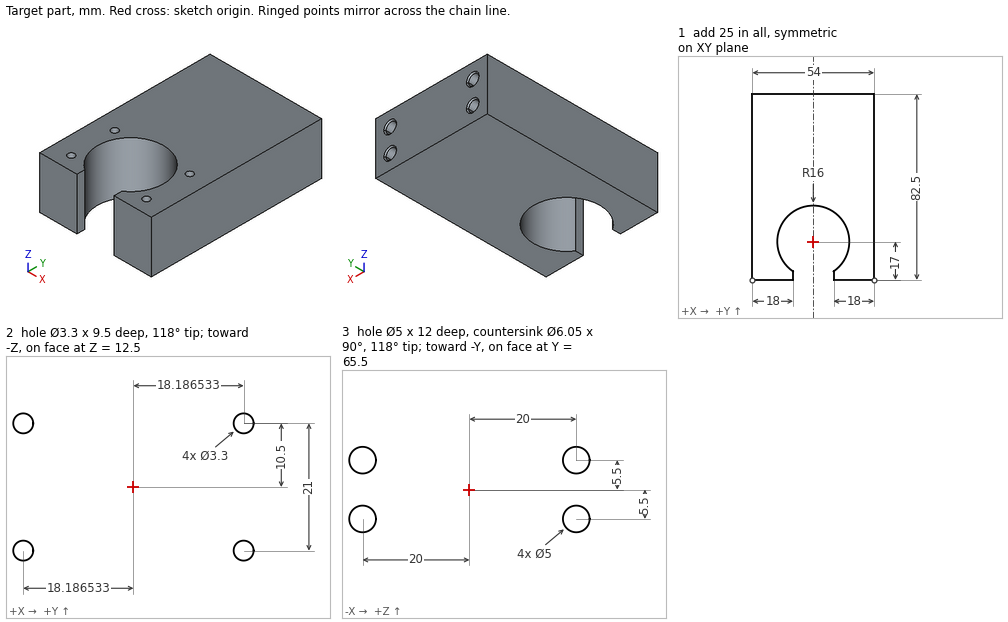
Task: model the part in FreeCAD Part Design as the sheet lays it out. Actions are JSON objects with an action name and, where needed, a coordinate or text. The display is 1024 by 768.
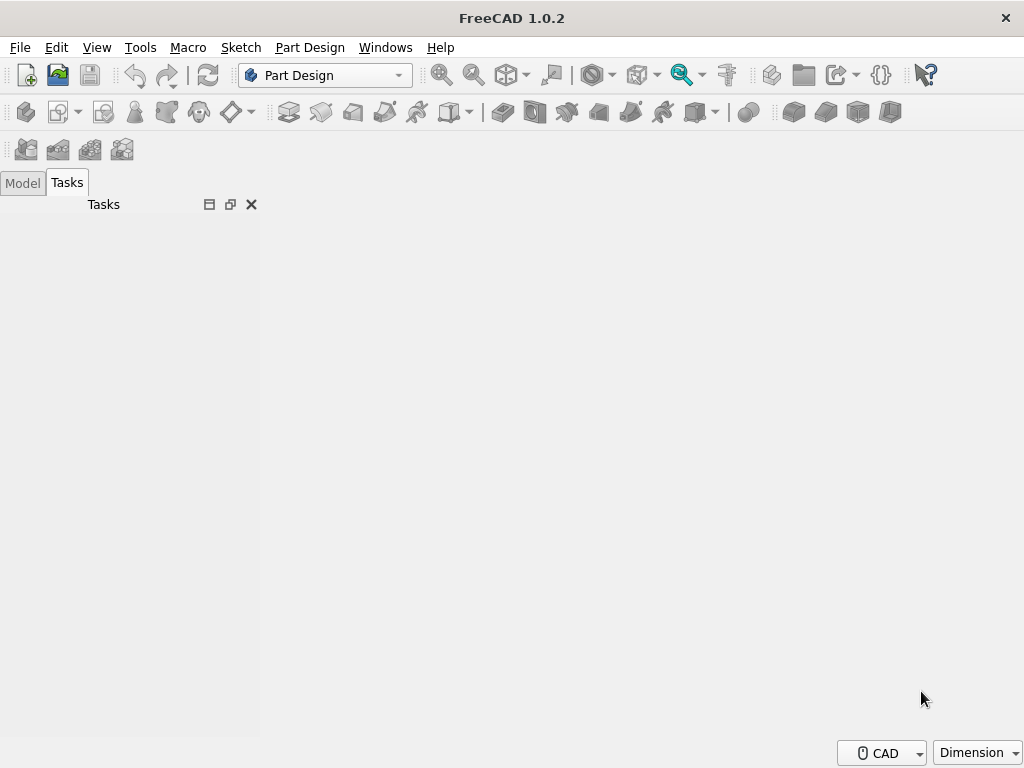
{"action": "left_click", "coordinate": [26, 76]}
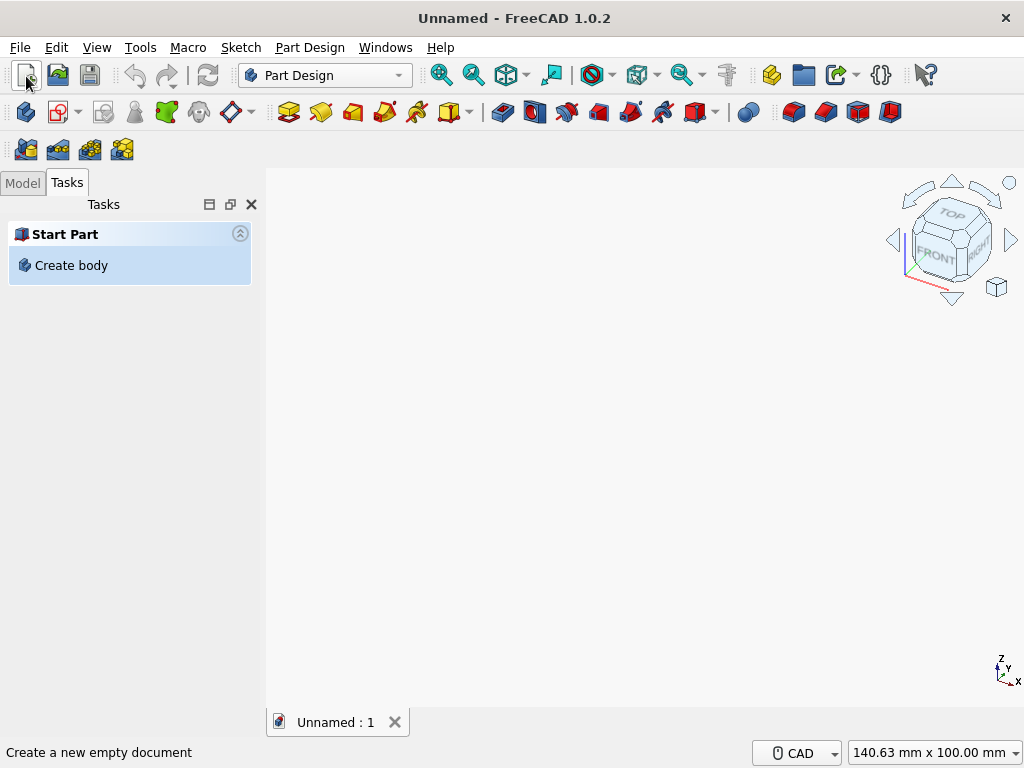
{"action": "left_click", "coordinate": [58, 112]}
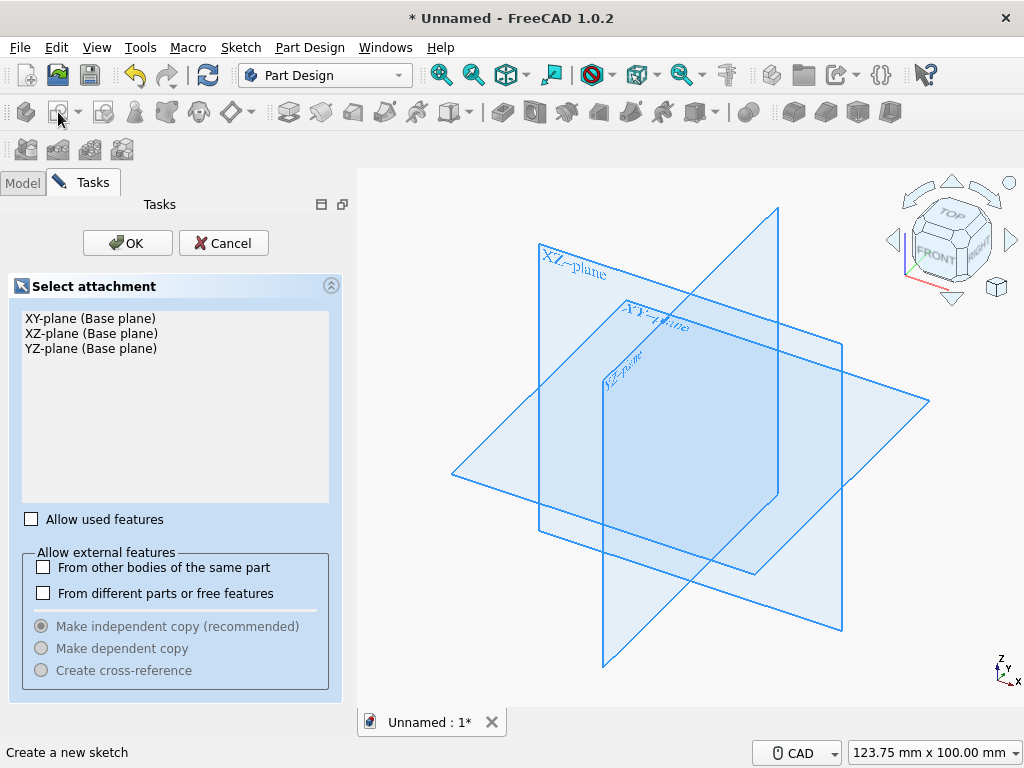
{"action": "left_click", "coordinate": [82, 318]}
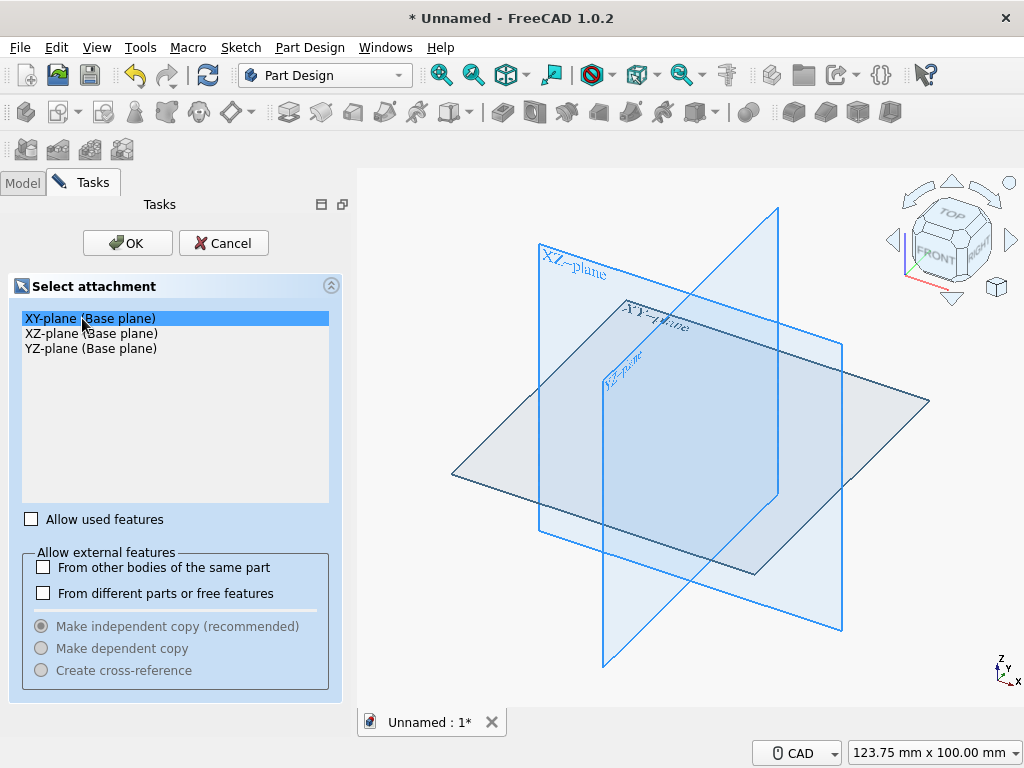
{"action": "left_click", "coordinate": [128, 243]}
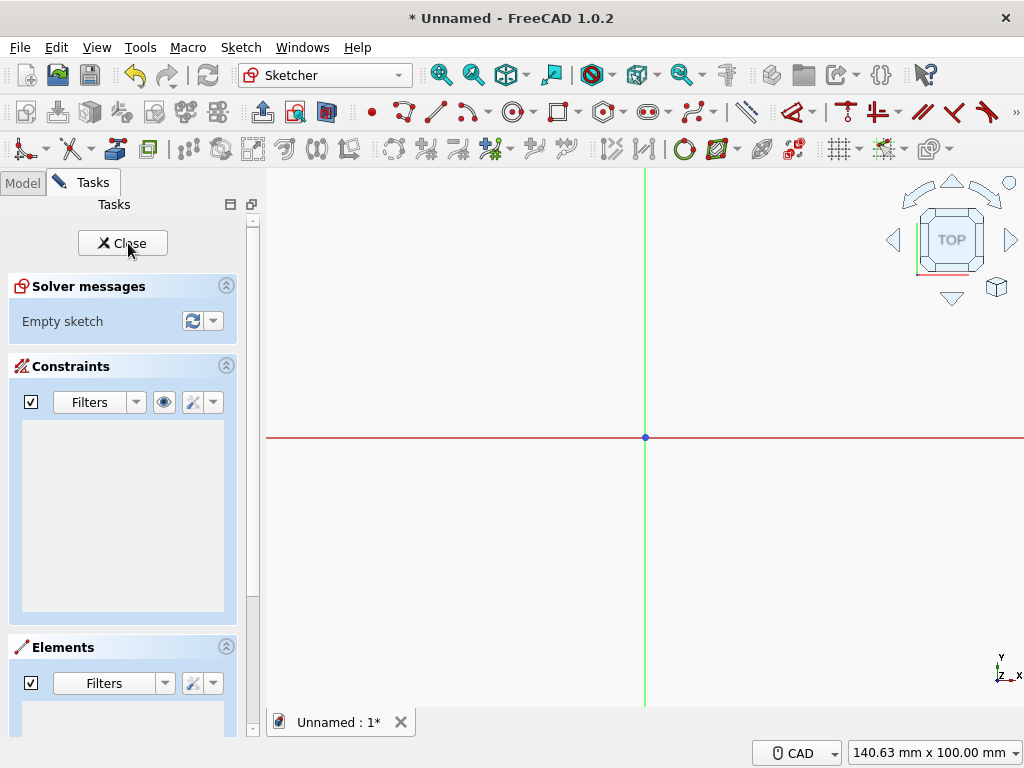
{"action": "scroll", "coordinate": [437, 679], "scroll_direction": "down", "scroll_amount": 2}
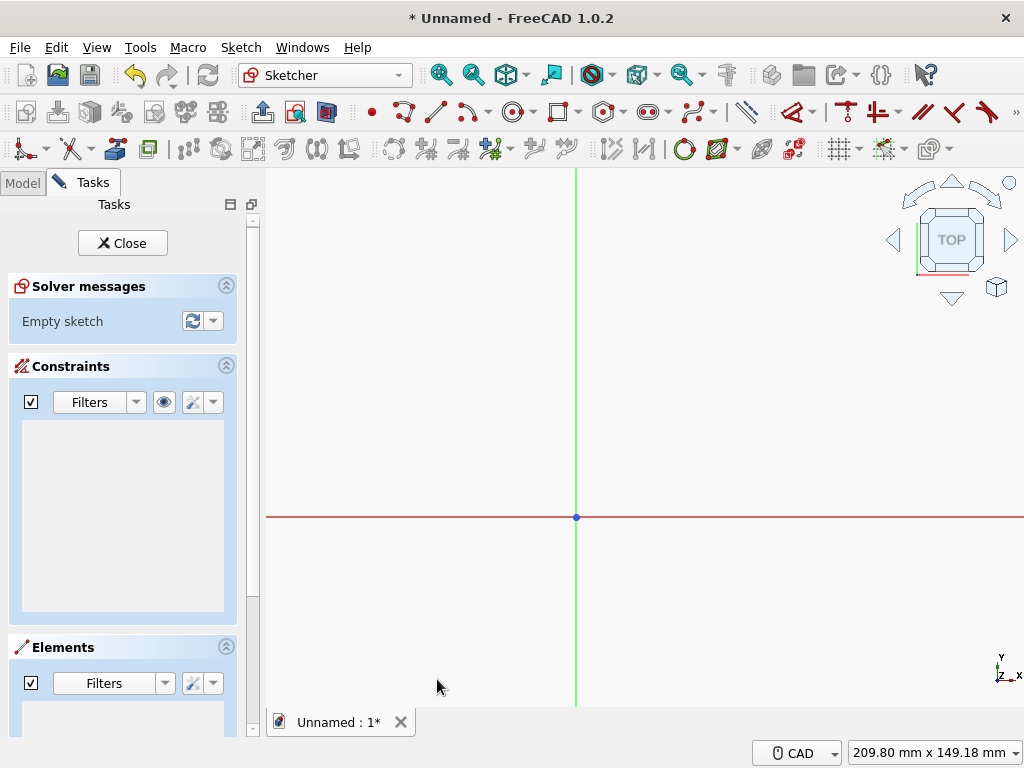
{"action": "left_click", "coordinate": [404, 112]}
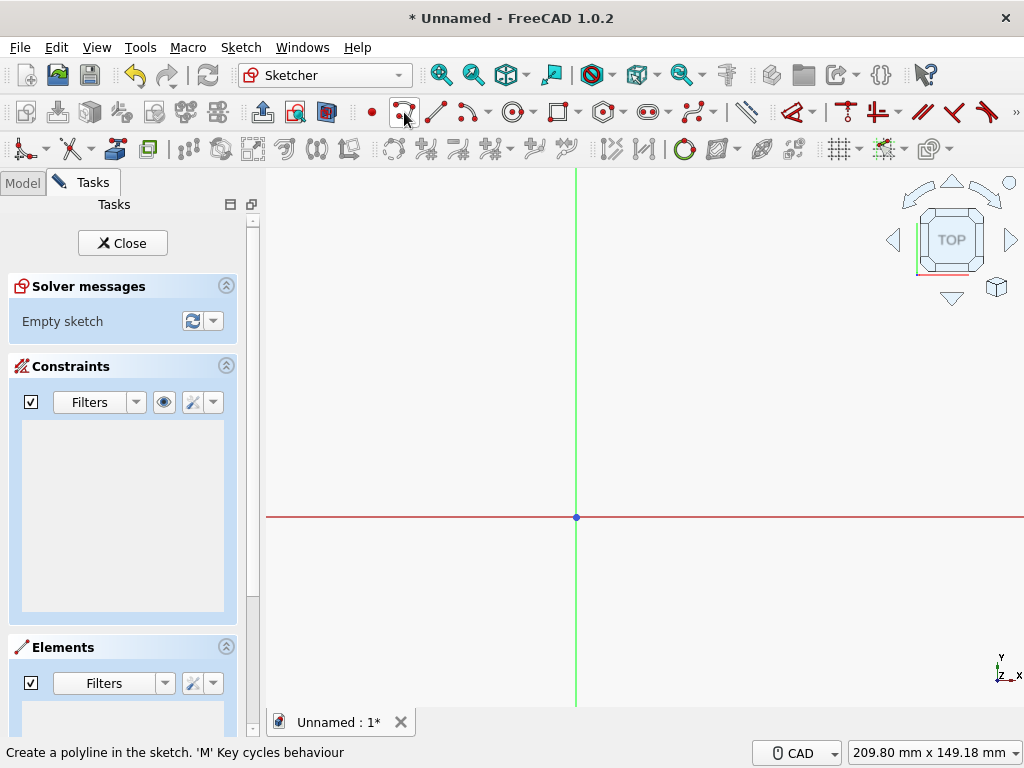
{"action": "left_click", "coordinate": [609, 565]}
{"action": "left_click", "coordinate": [609, 579]}
{"action": "left_click", "coordinate": [674, 579]}
{"action": "left_click", "coordinate": [674, 281]}
{"action": "left_click", "coordinate": [479, 281]}
{"action": "left_click", "coordinate": [479, 579]}
{"action": "left_click", "coordinate": [544, 579]}
{"action": "left_click", "coordinate": [544, 565]}
{"action": "right_click", "coordinate": [544, 565]}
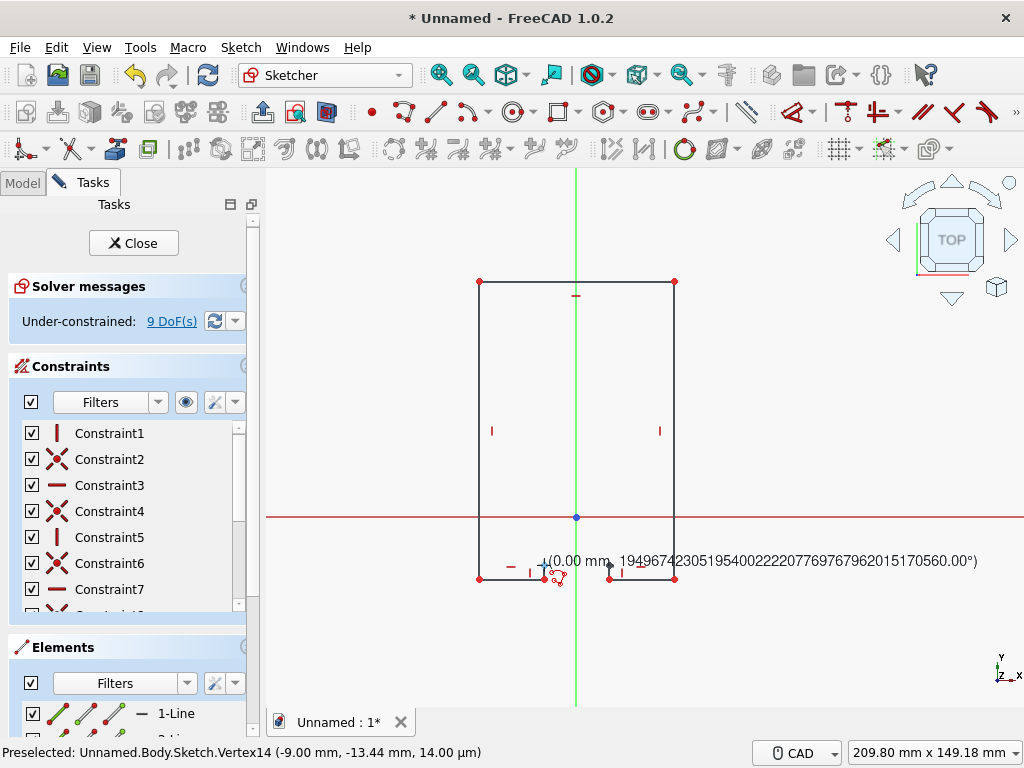
{"action": "key", "text": "g 3 a"}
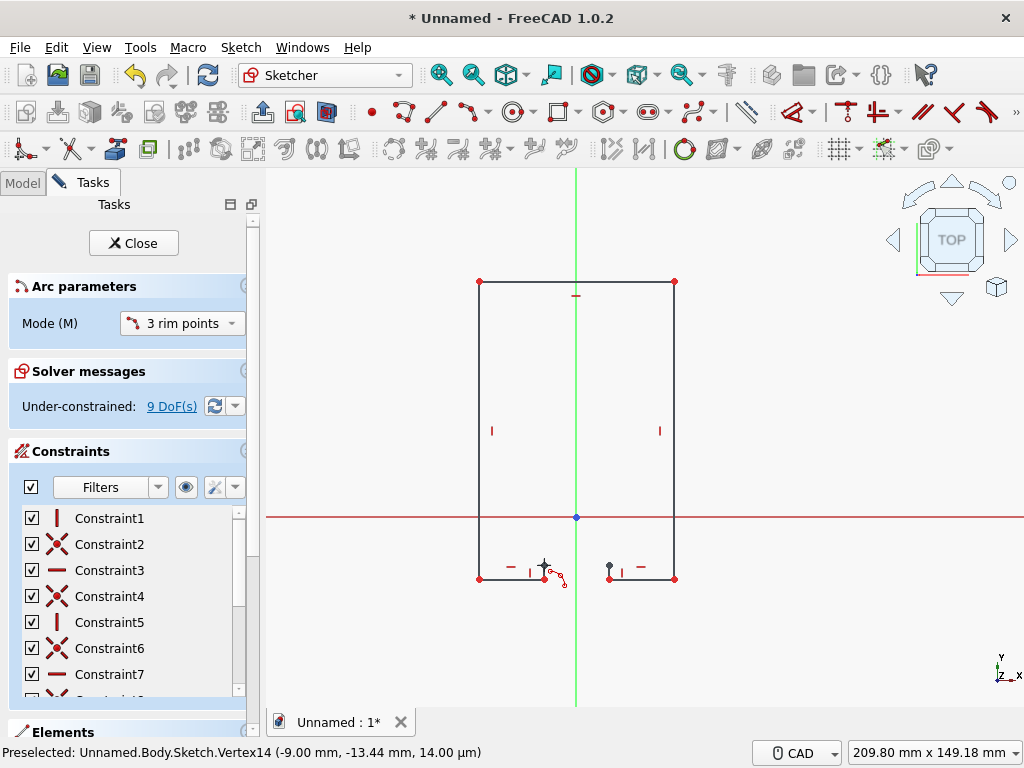
{"action": "scroll", "coordinate": [544, 565], "scroll_direction": "up", "scroll_amount": 5}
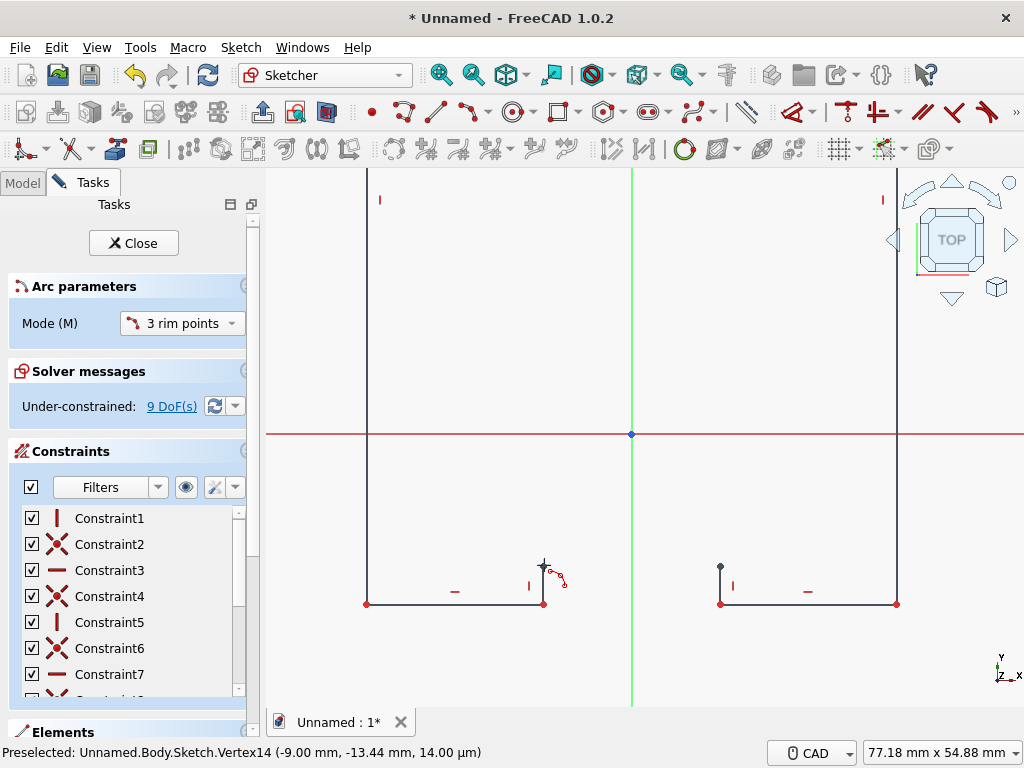
{"action": "left_click", "coordinate": [543, 566]}
{"action": "left_click", "coordinate": [720, 566]}
{"action": "left_click", "coordinate": [708, 297]}
{"action": "key", "text": "Escape"}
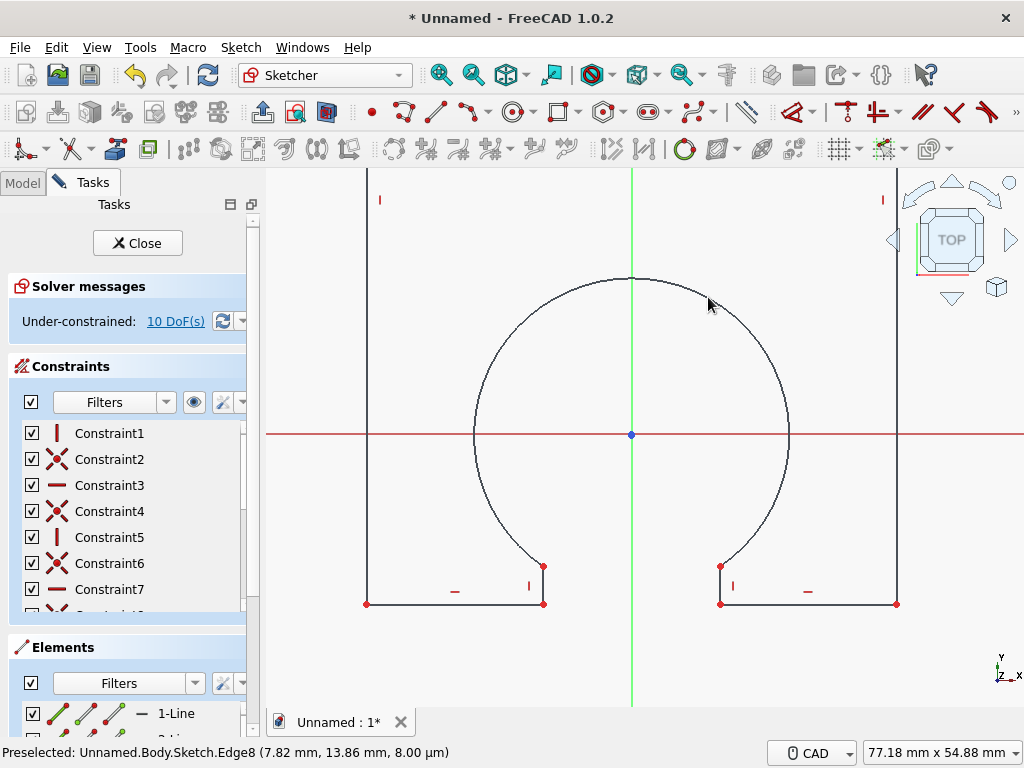
{"action": "left_click_drag", "start_coordinate": [622, 424], "coordinate": [642, 446]}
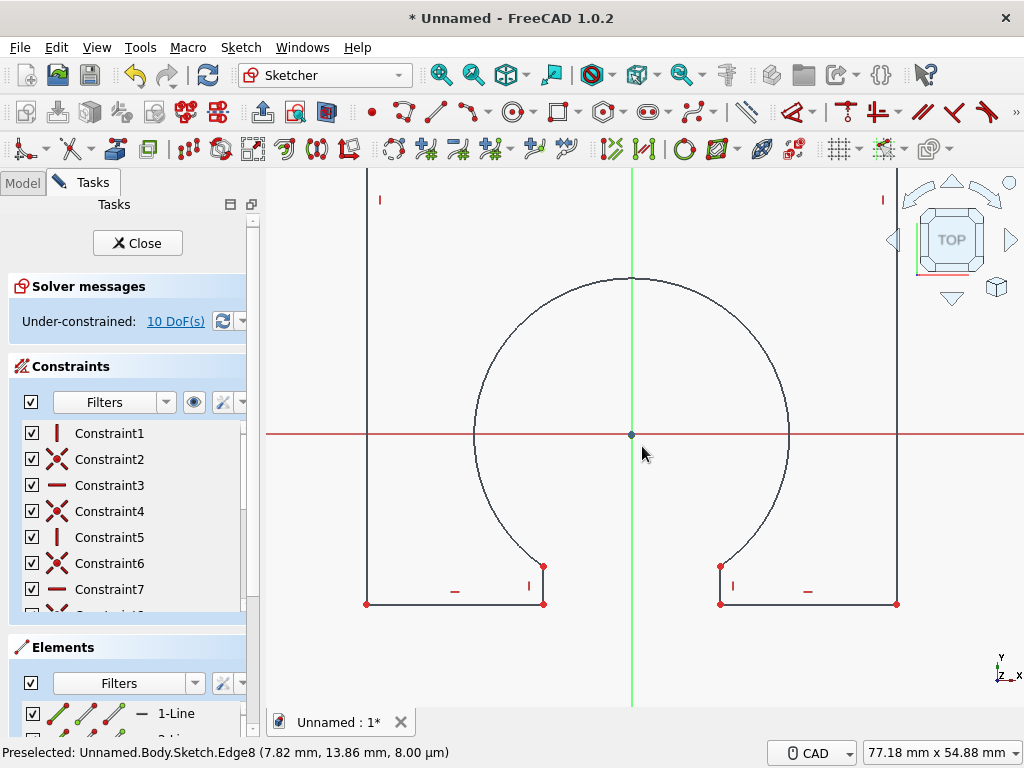
{"action": "left_click", "coordinate": [846, 112]}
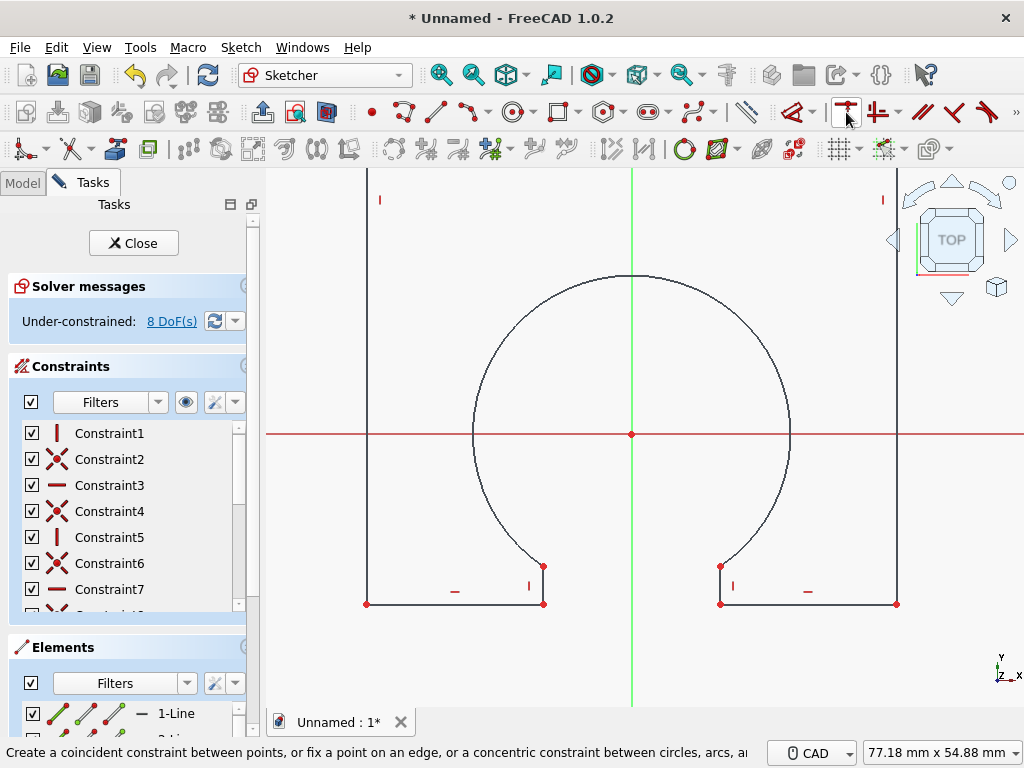
{"action": "scroll", "coordinate": [531, 634], "scroll_direction": "down", "scroll_amount": 4}